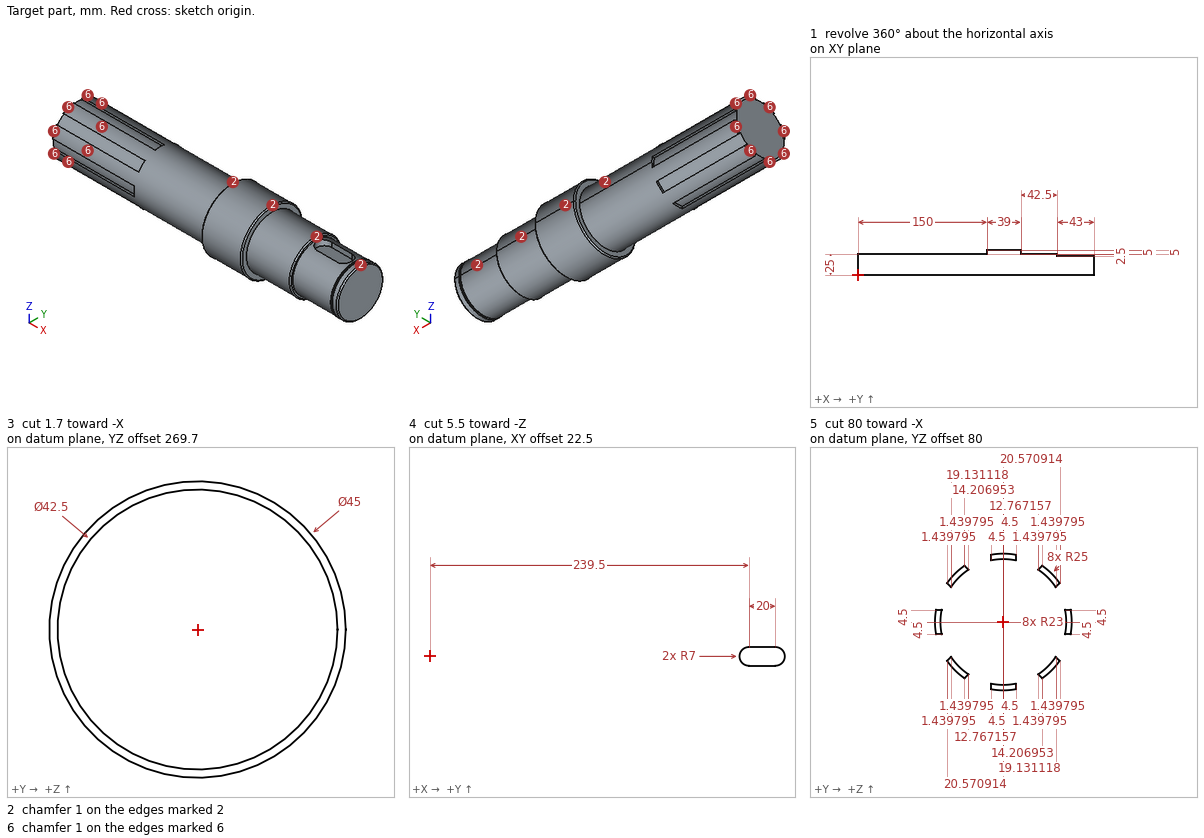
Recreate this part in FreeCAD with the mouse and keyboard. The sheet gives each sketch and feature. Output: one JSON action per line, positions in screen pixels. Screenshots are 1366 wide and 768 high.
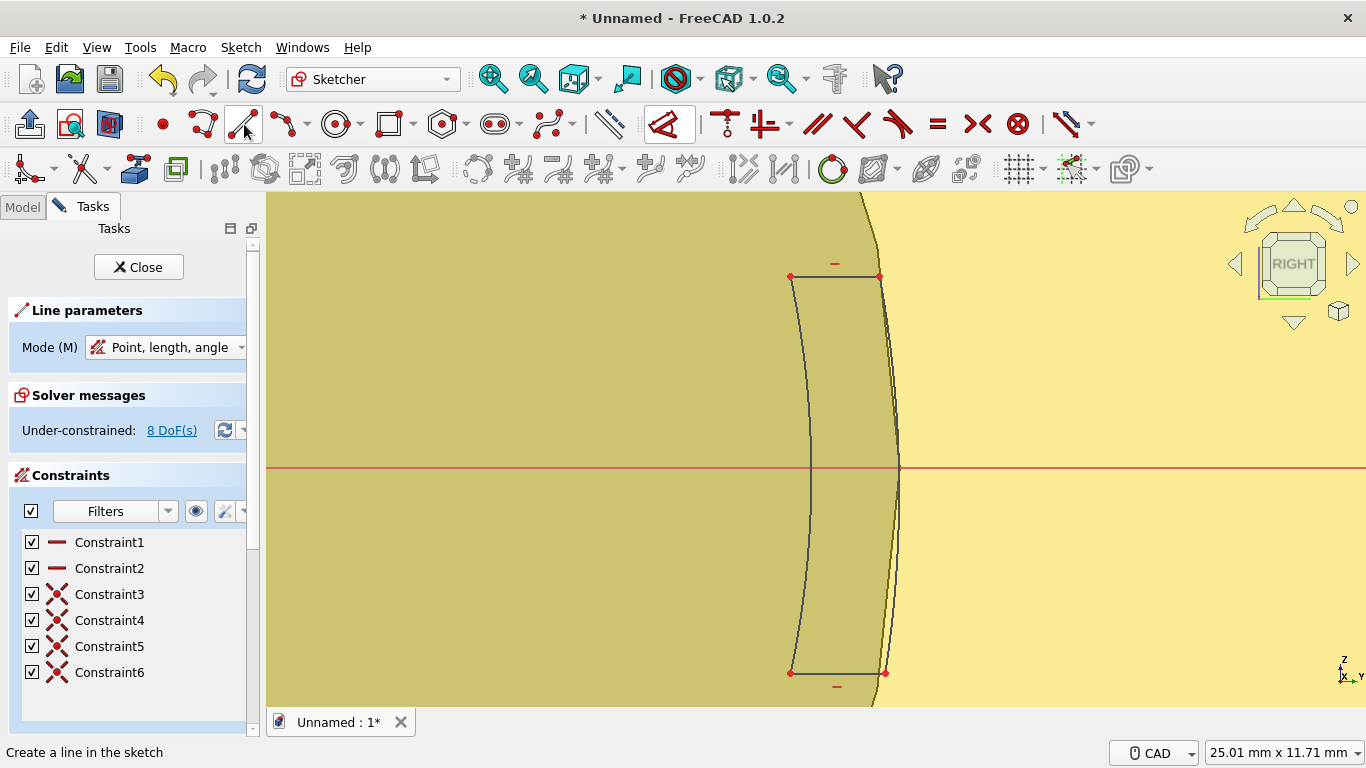
{"action": "scroll", "coordinate": [896, 447], "scroll_direction": "down", "scroll_amount": 10}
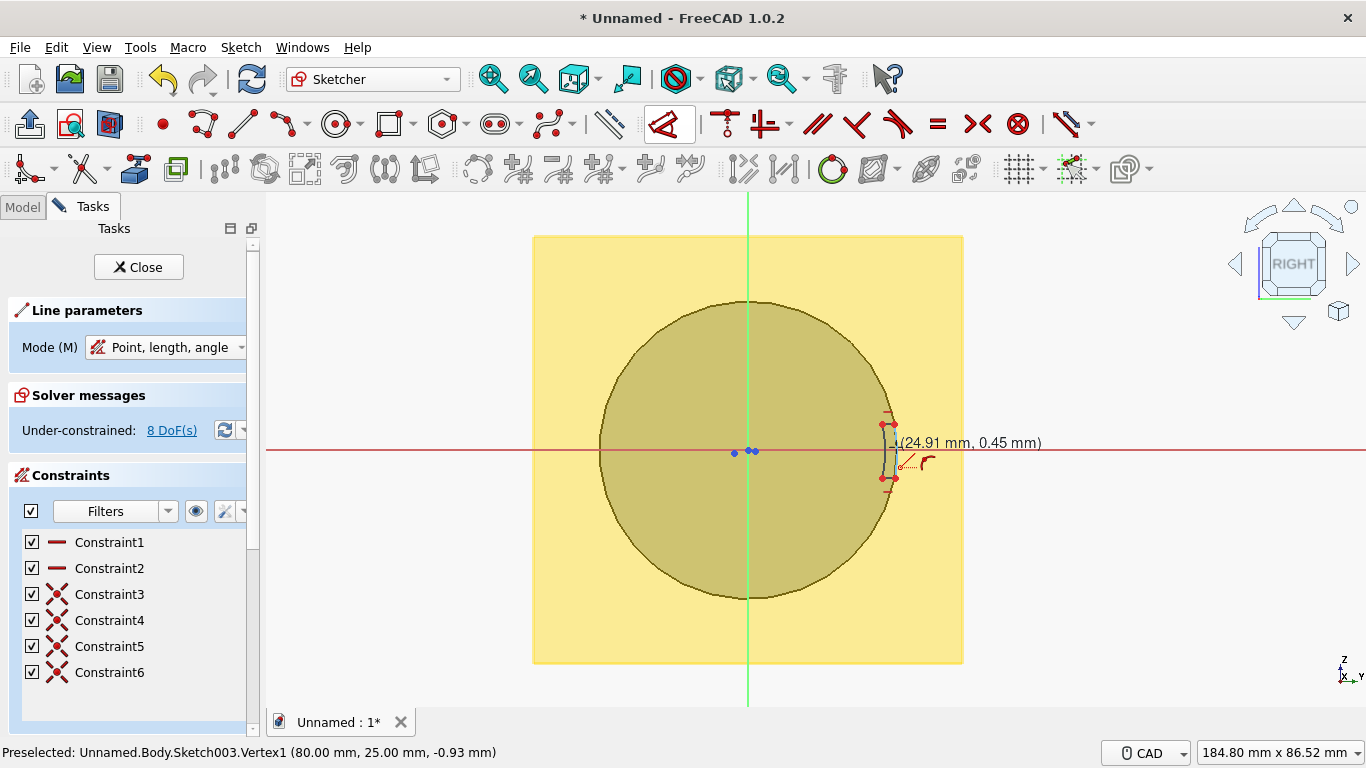
{"action": "left_click", "coordinate": [824, 336]}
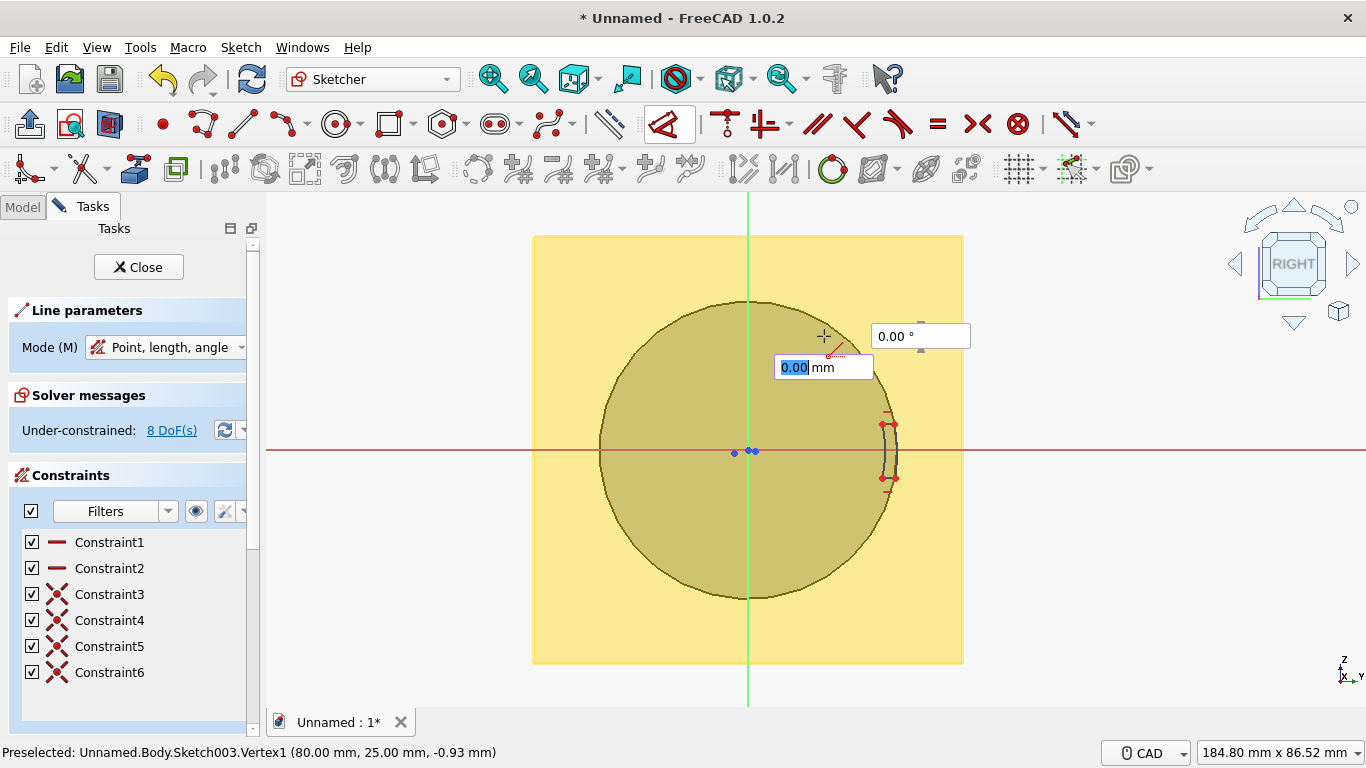
{"action": "scroll", "coordinate": [833, 328], "scroll_direction": "up", "scroll_amount": 2}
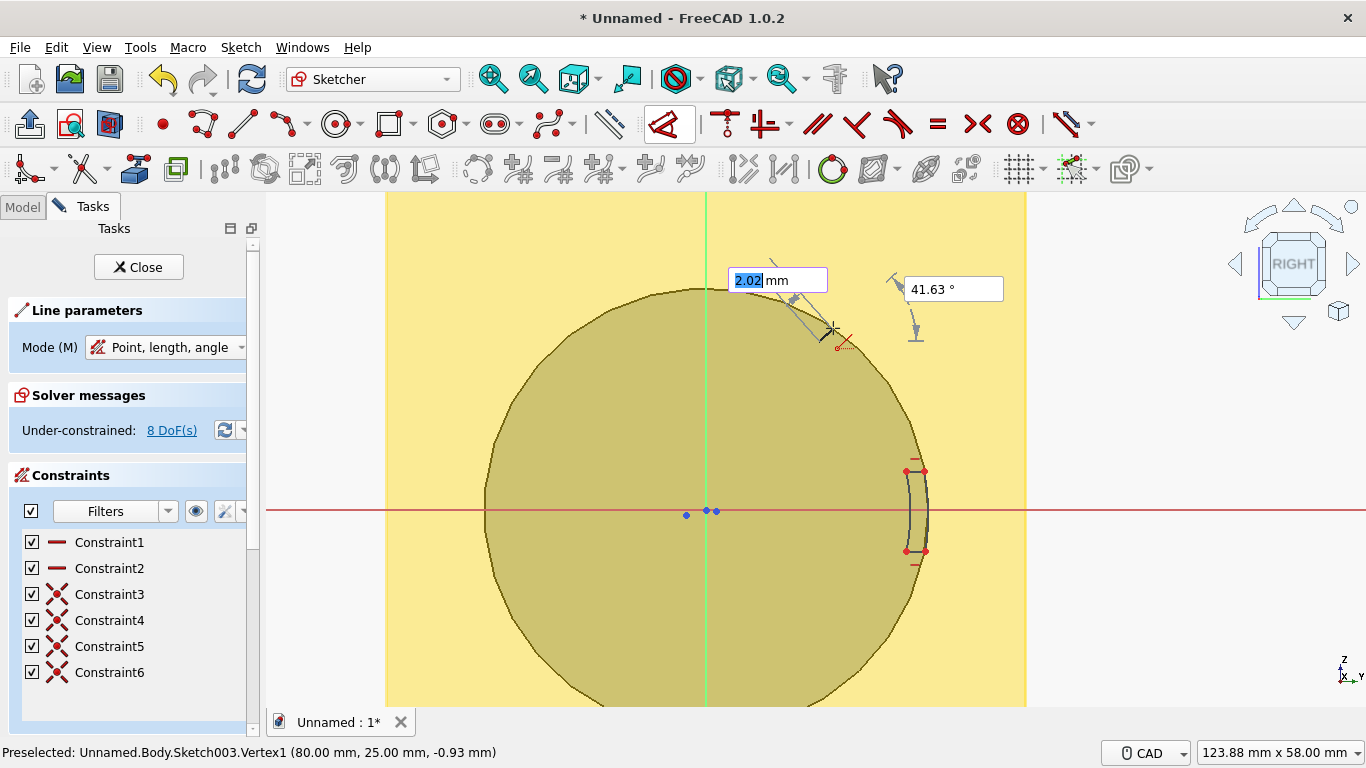
{"action": "left_click", "coordinate": [832, 328]}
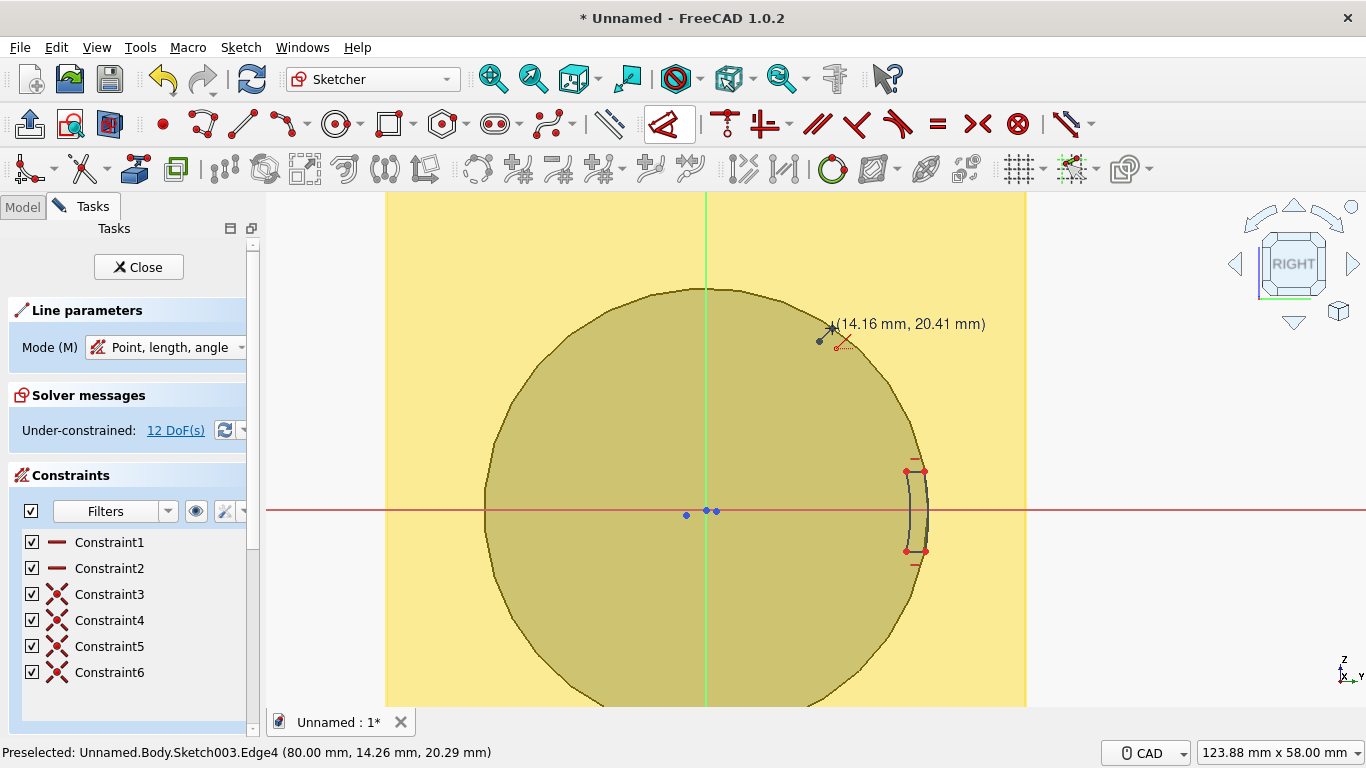
{"action": "left_click", "coordinate": [889, 384]}
{"action": "left_click", "coordinate": [876, 397]}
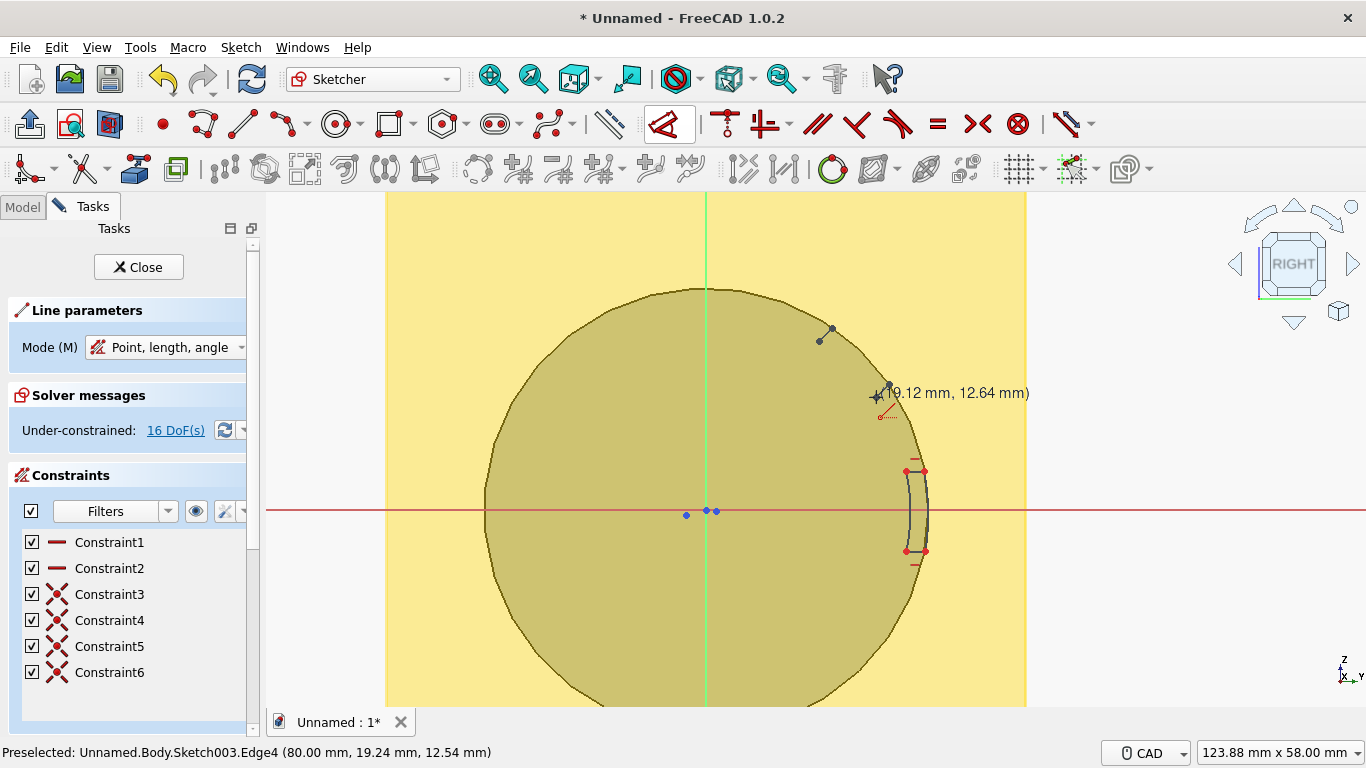
{"action": "left_click", "coordinate": [284, 124]}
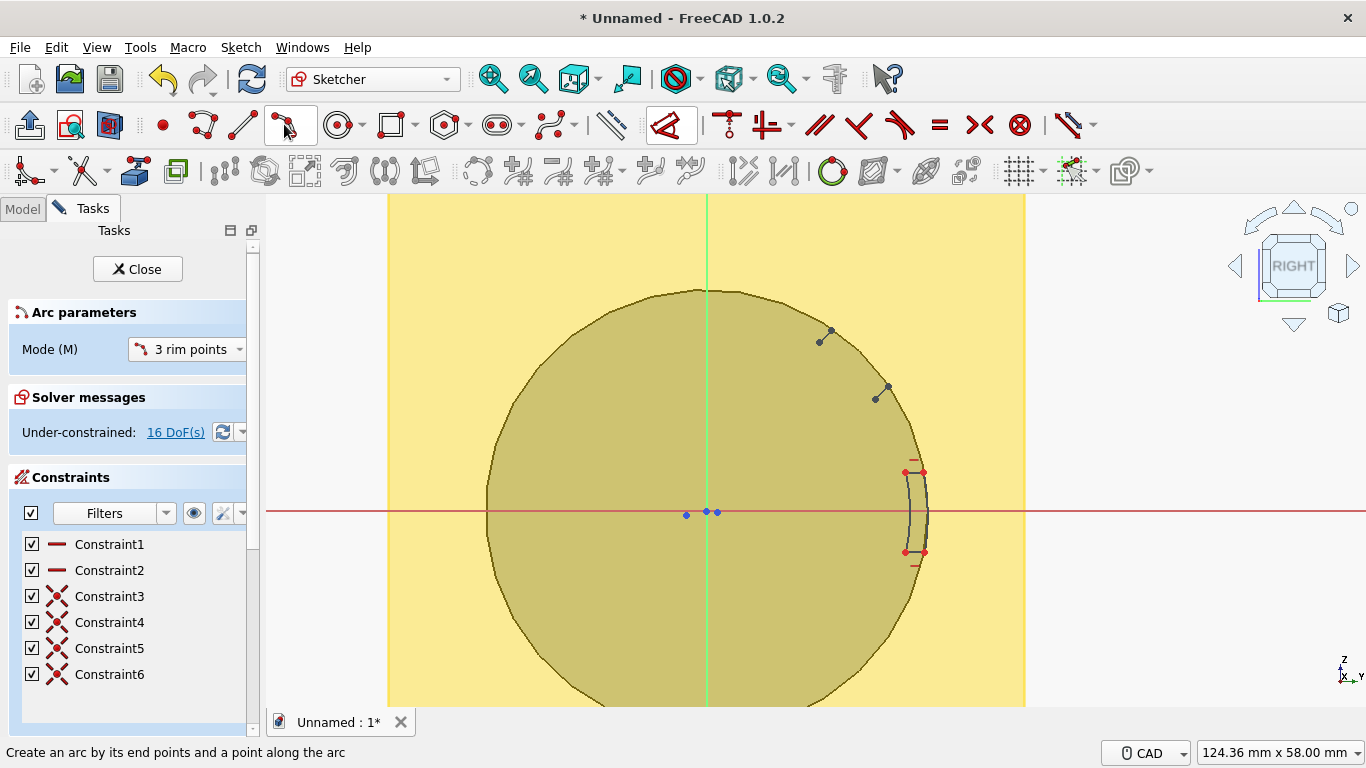
{"action": "scroll", "coordinate": [832, 329], "scroll_direction": "up", "scroll_amount": 3}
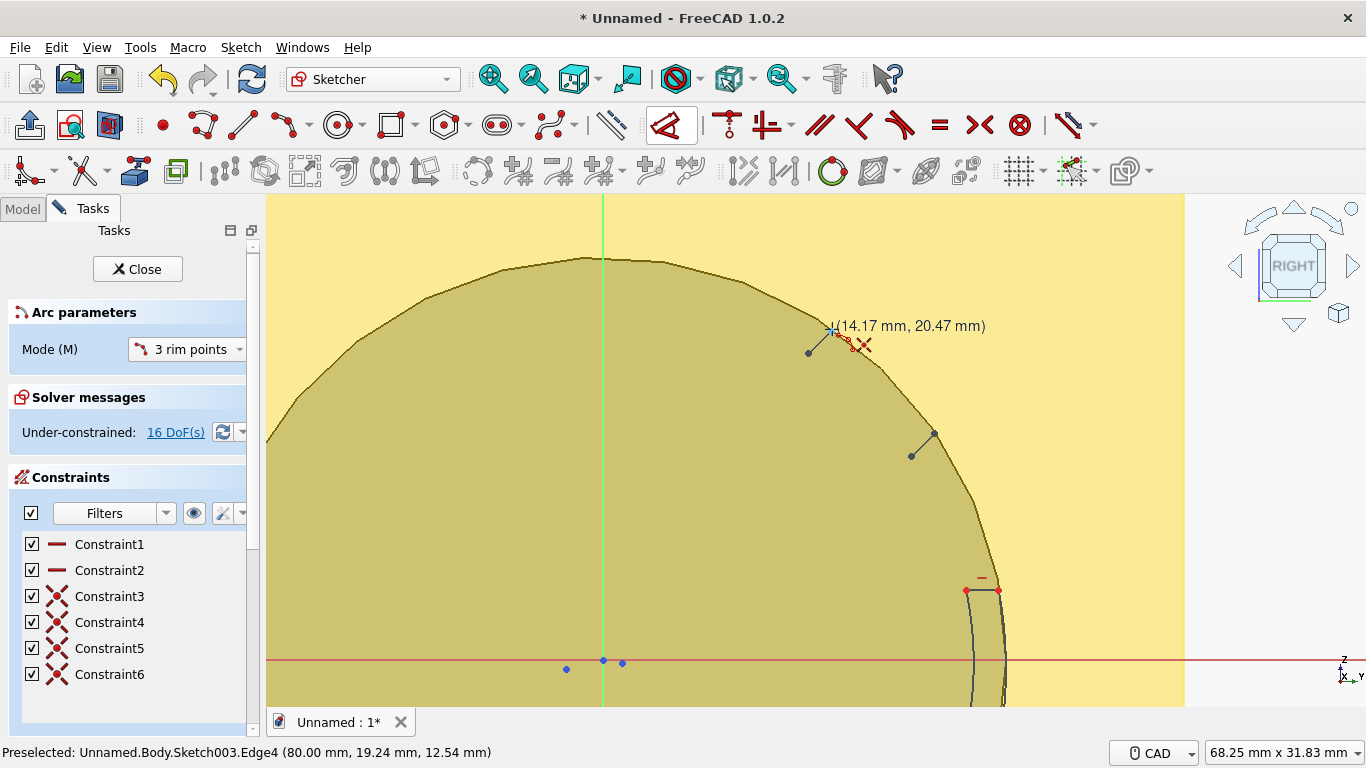
{"action": "left_click", "coordinate": [831, 331]}
{"action": "left_click", "coordinate": [935, 433]}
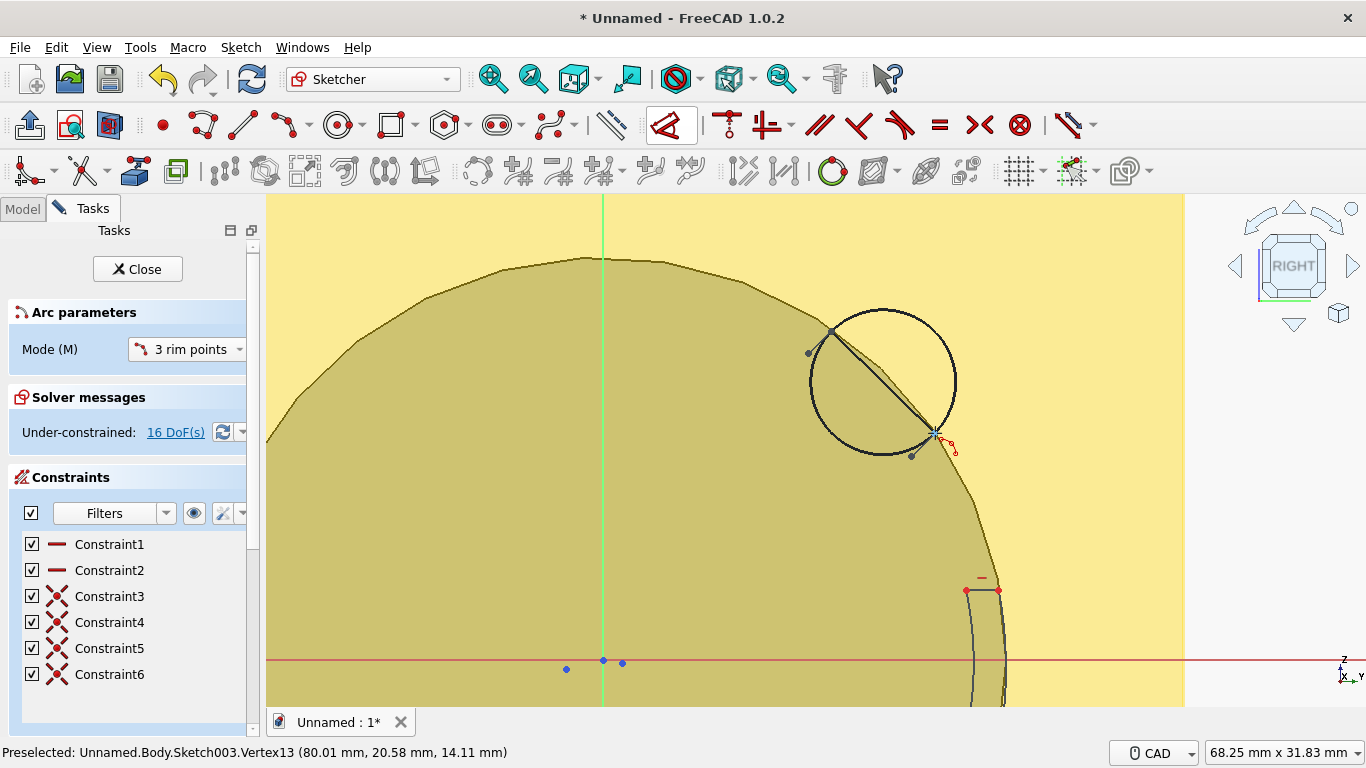
{"action": "scroll", "coordinate": [888, 376], "scroll_direction": "up", "scroll_amount": 5}